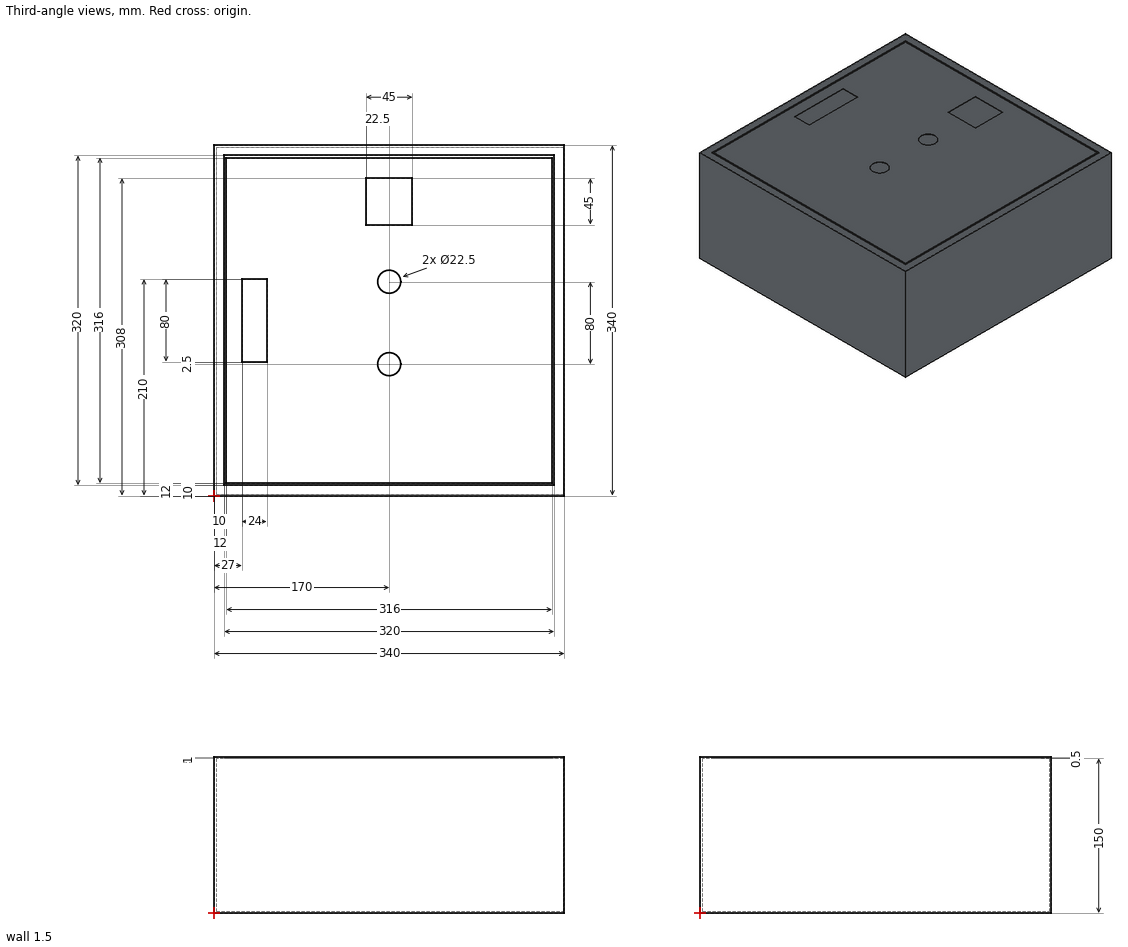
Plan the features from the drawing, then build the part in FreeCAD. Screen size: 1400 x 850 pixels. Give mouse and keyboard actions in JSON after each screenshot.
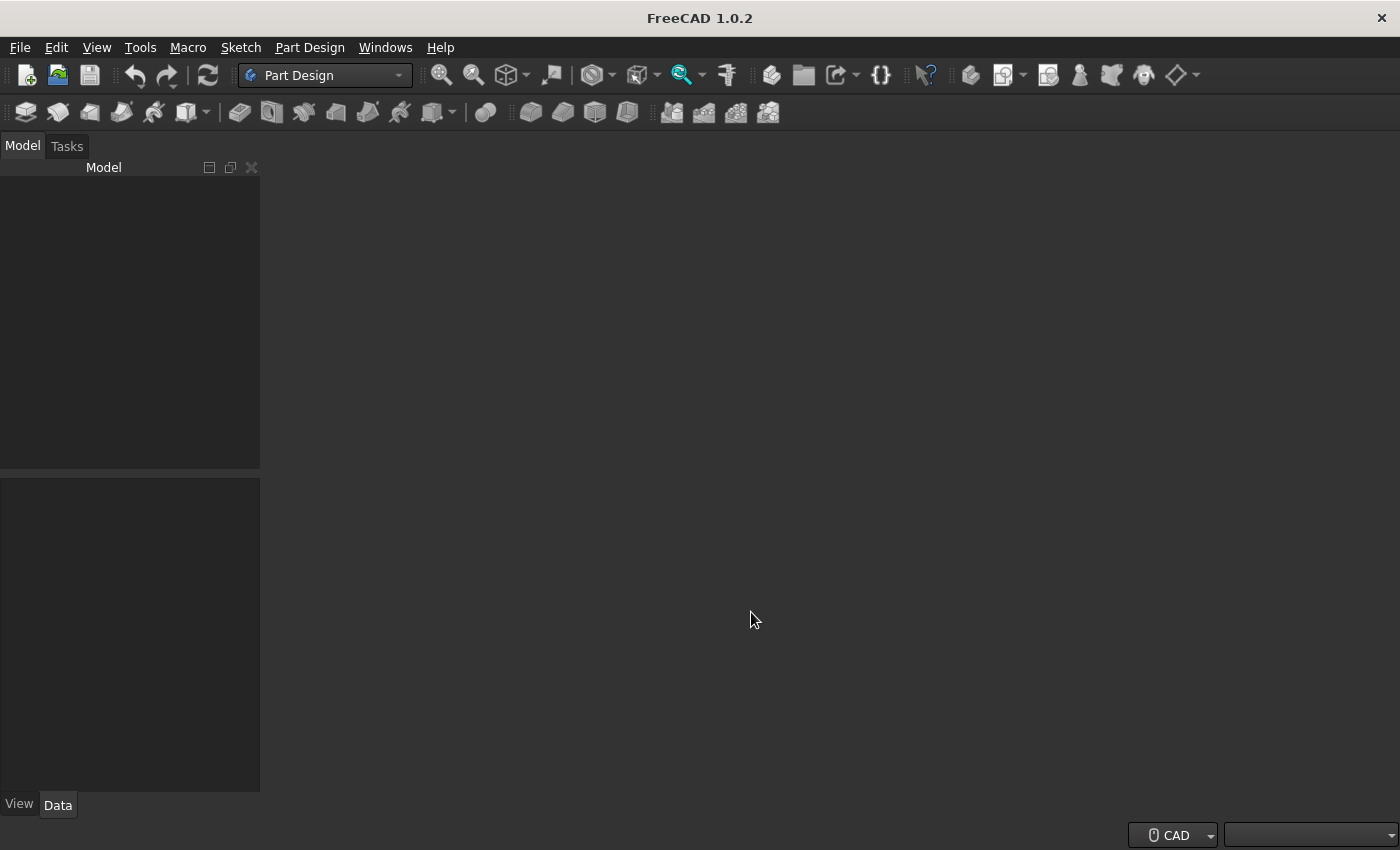
{"action": "left_click", "coordinate": [26, 76]}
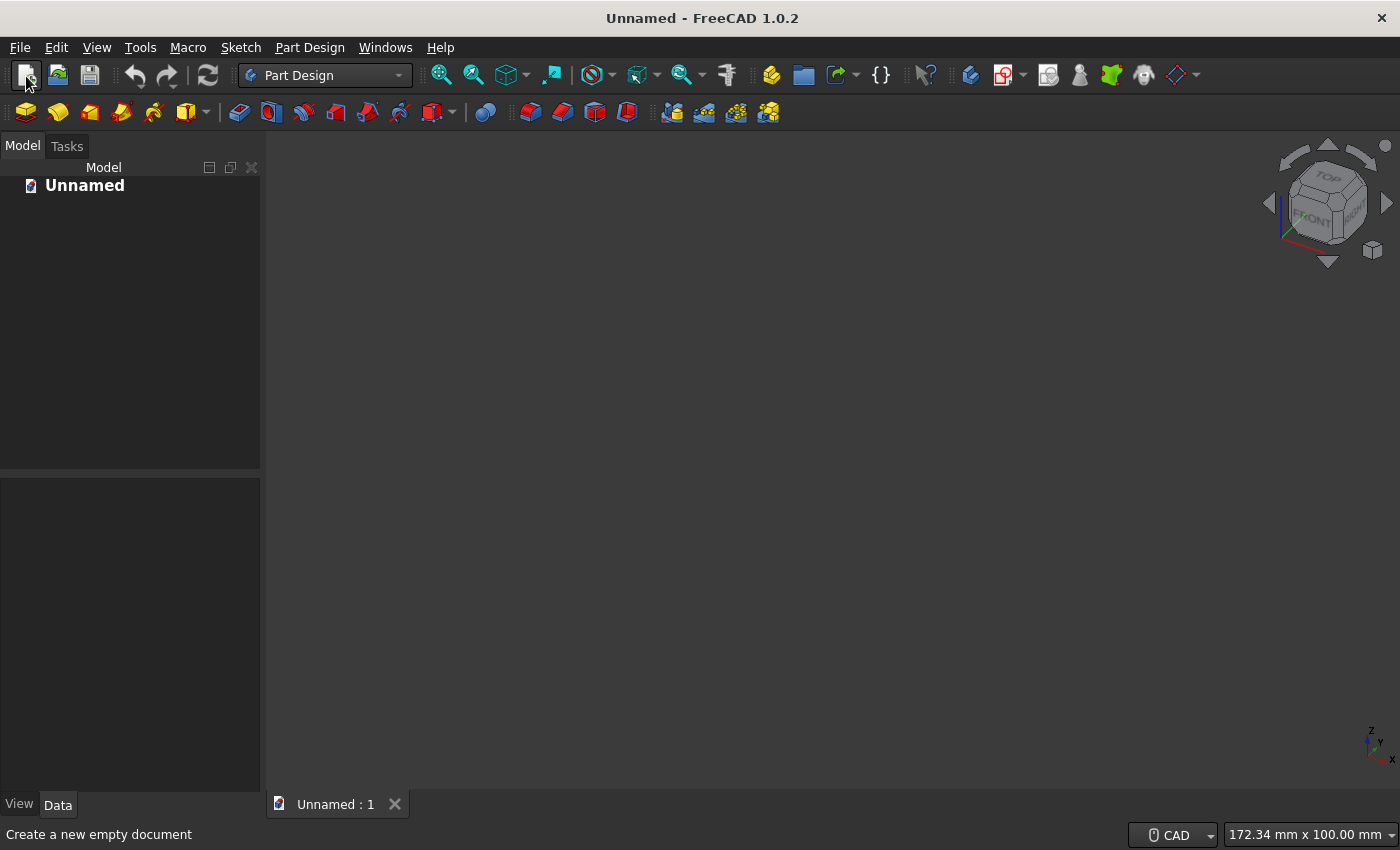
{"action": "left_click", "coordinate": [1004, 76]}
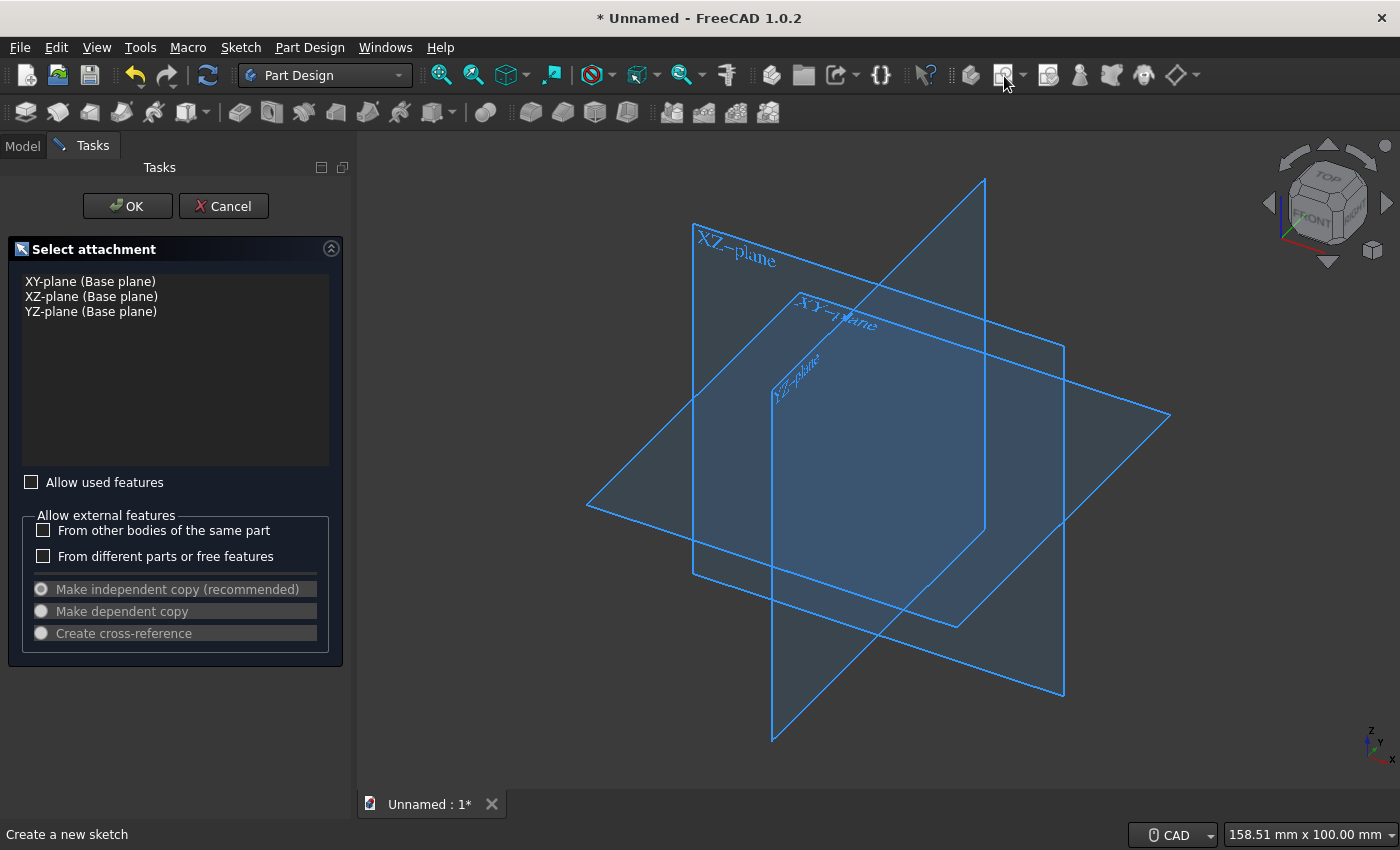
{"action": "left_click", "coordinate": [82, 282]}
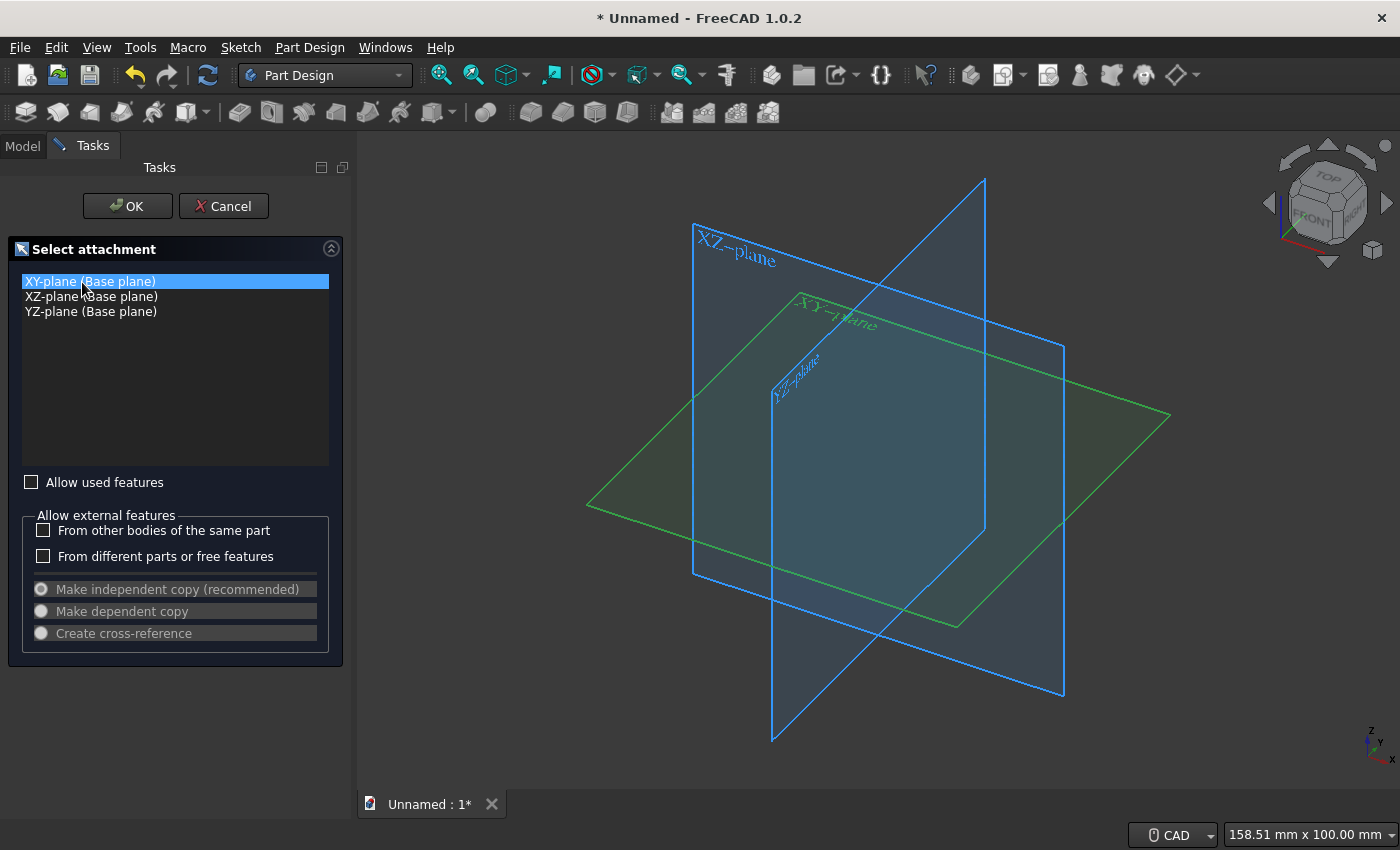
{"action": "left_click", "coordinate": [128, 206]}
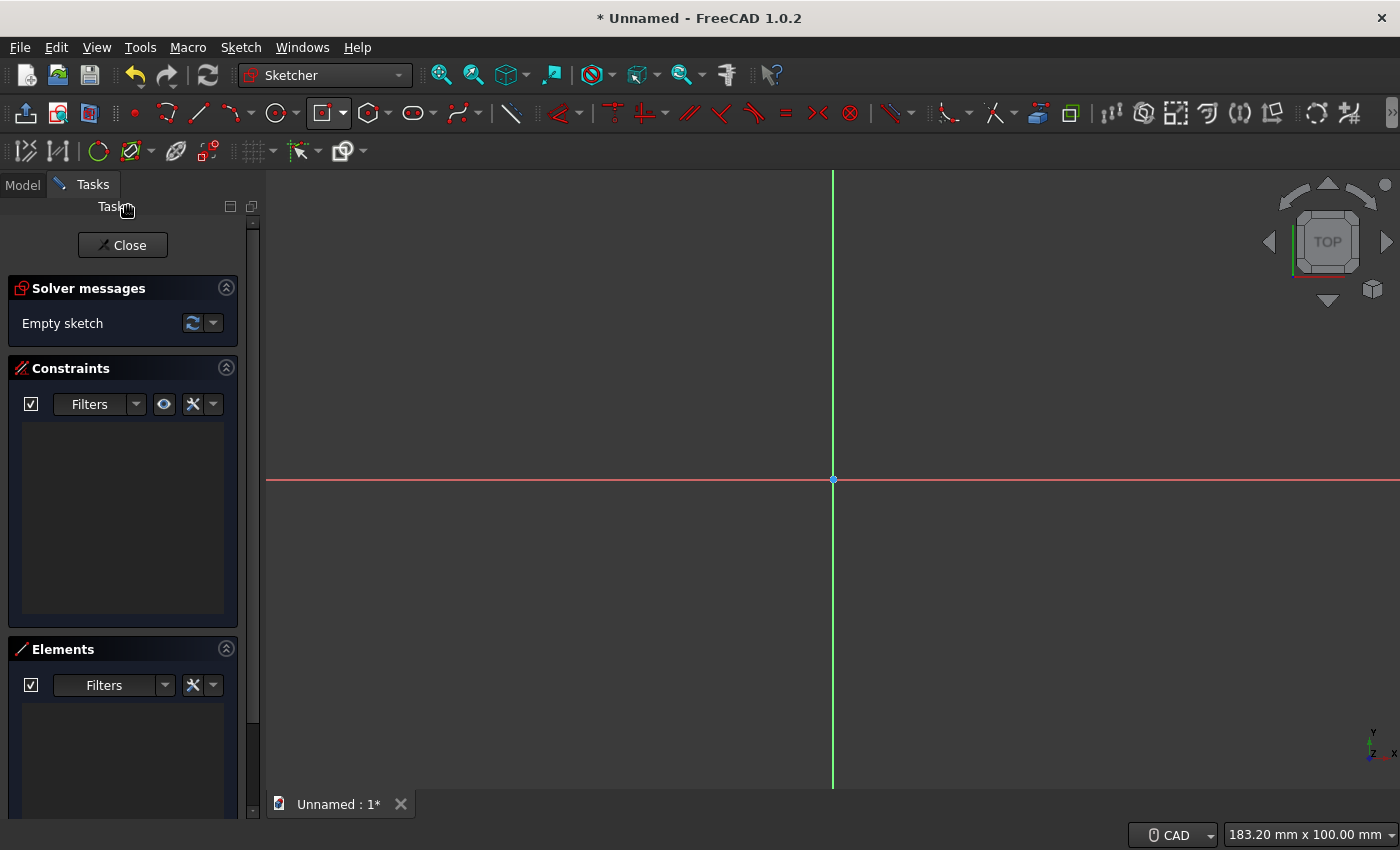
{"action": "scroll", "coordinate": [481, 746], "scroll_direction": "down", "scroll_amount": 8}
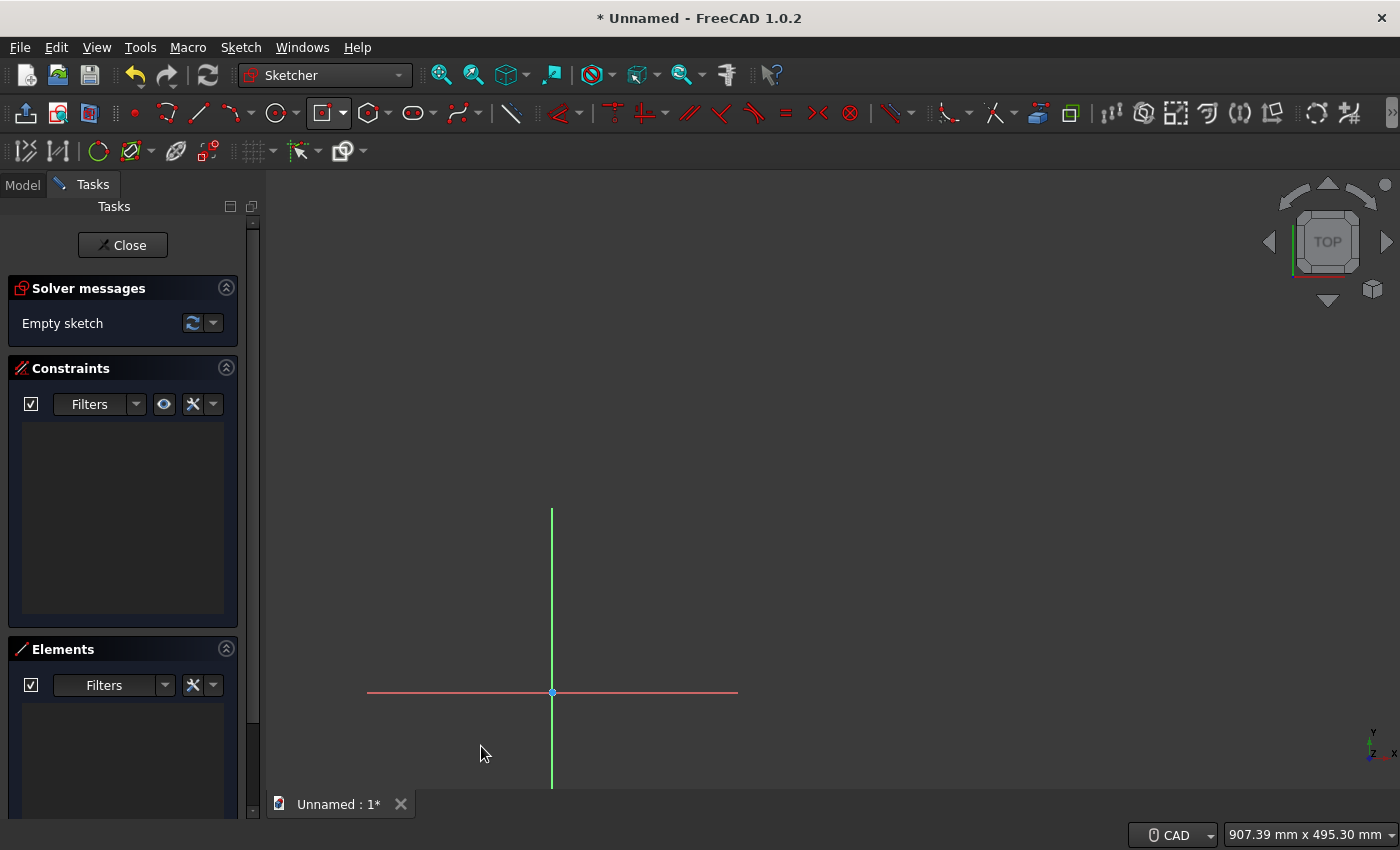
{"action": "key", "text": "g r"}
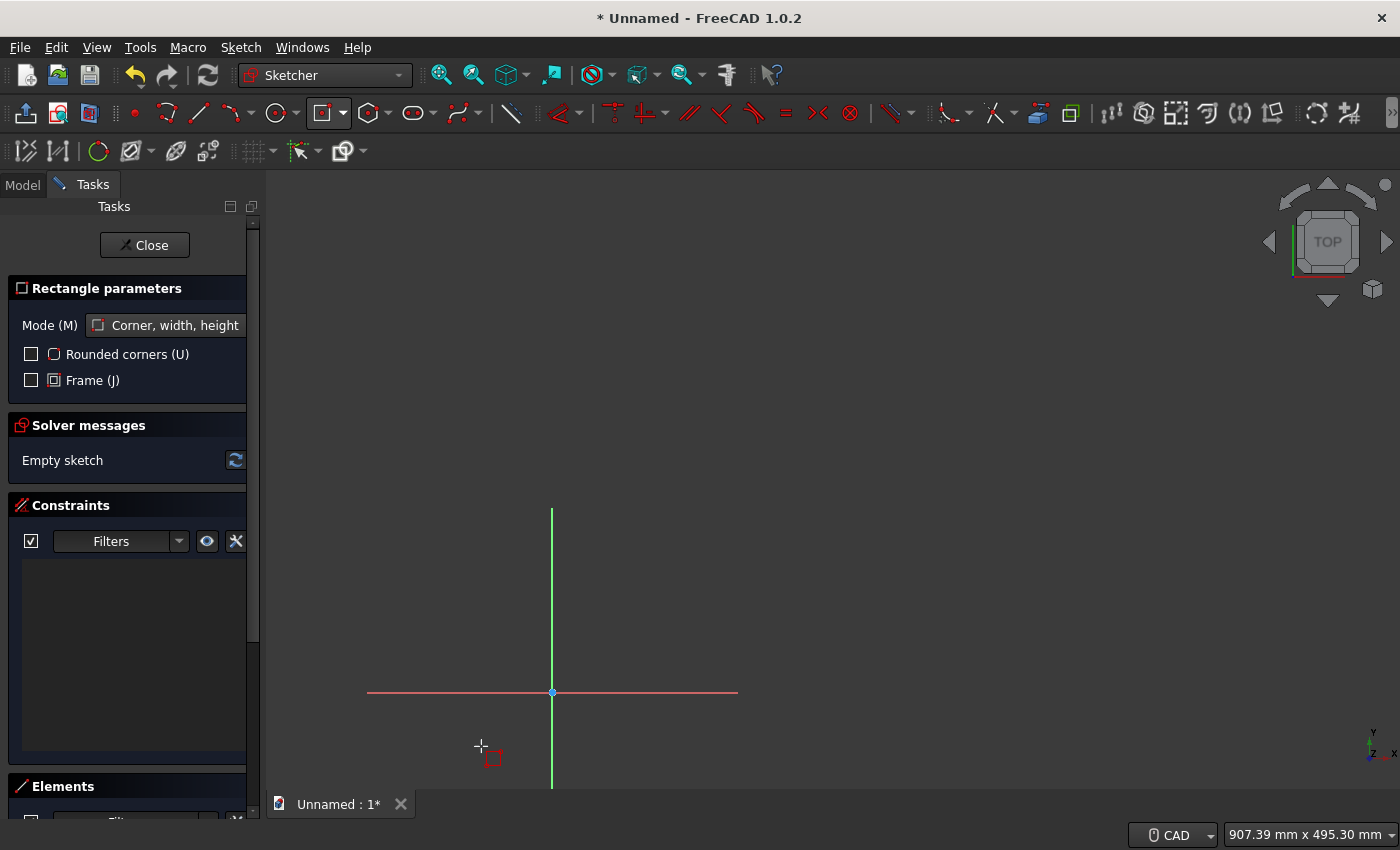
{"action": "left_click", "coordinate": [552, 693]}
{"action": "mouse_move", "coordinate": [977, 268]}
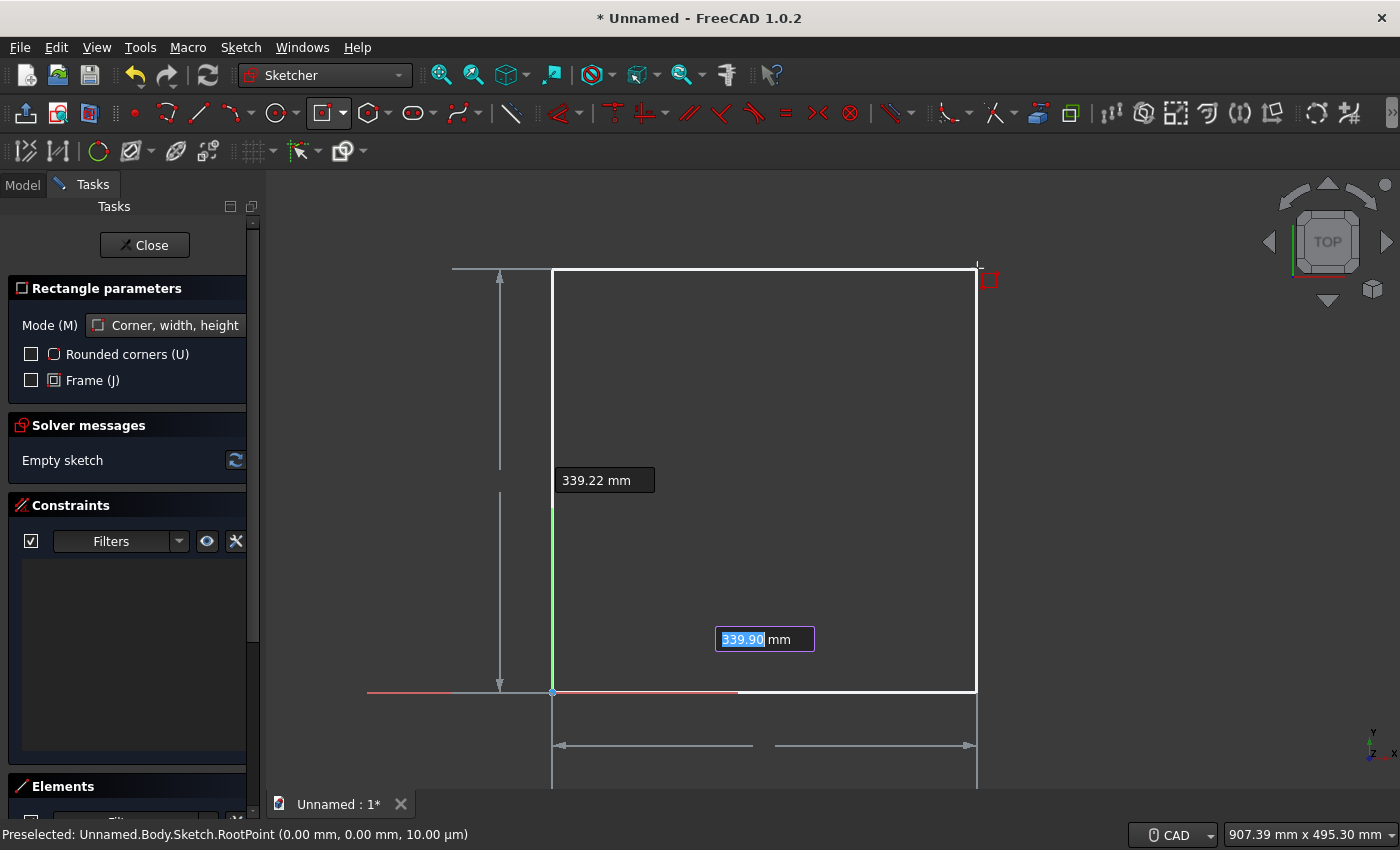
{"action": "type", "text": "340"}
{"action": "key", "text": "Tab"}
{"action": "type", "text": "340"}
{"action": "key", "text": "Return"}
{"action": "key", "text": "Escape"}